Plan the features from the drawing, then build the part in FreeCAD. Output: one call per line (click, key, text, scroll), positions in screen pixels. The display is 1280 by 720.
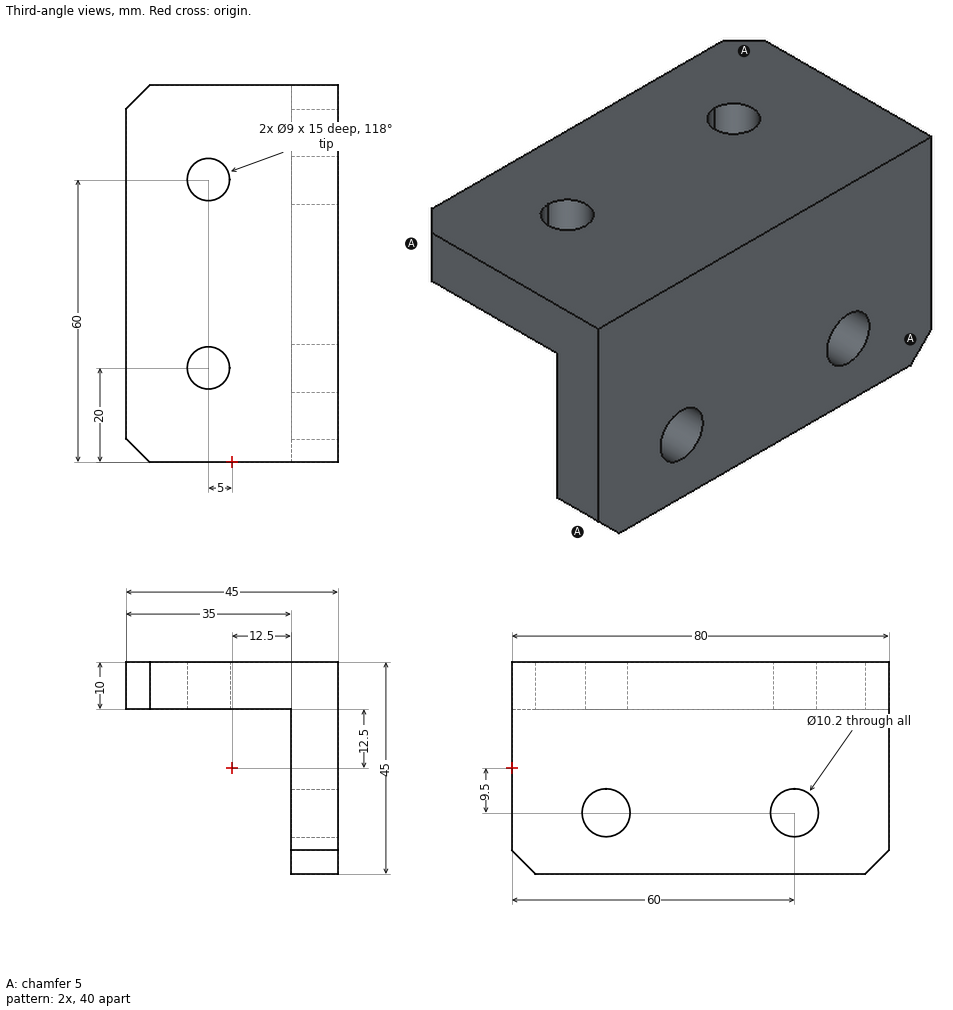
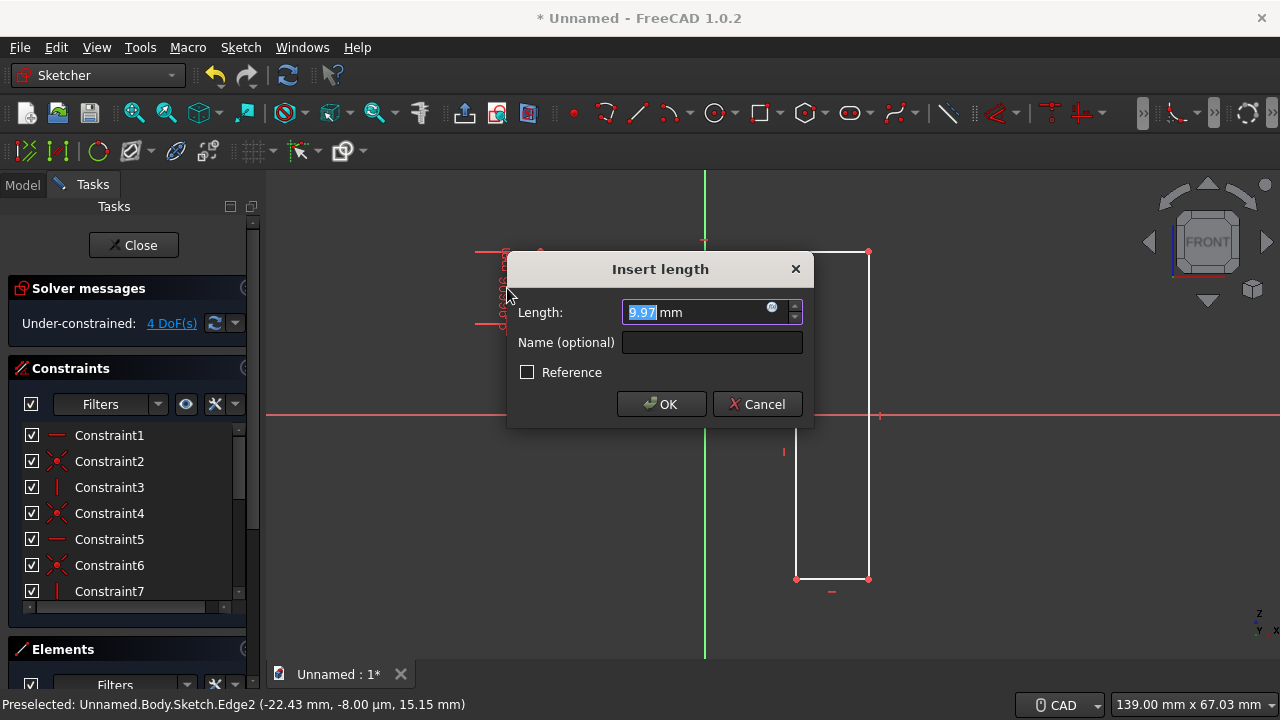
text(10)
key(Return)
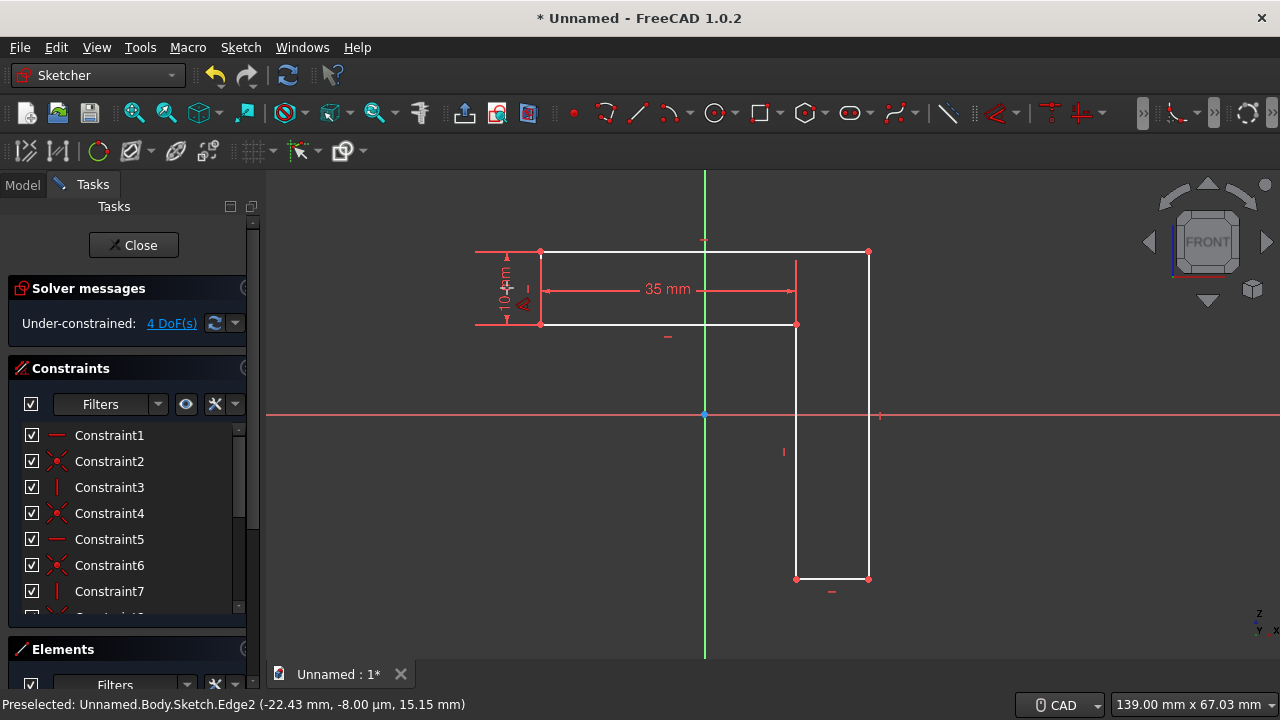
click(639, 252)
click(629, 218)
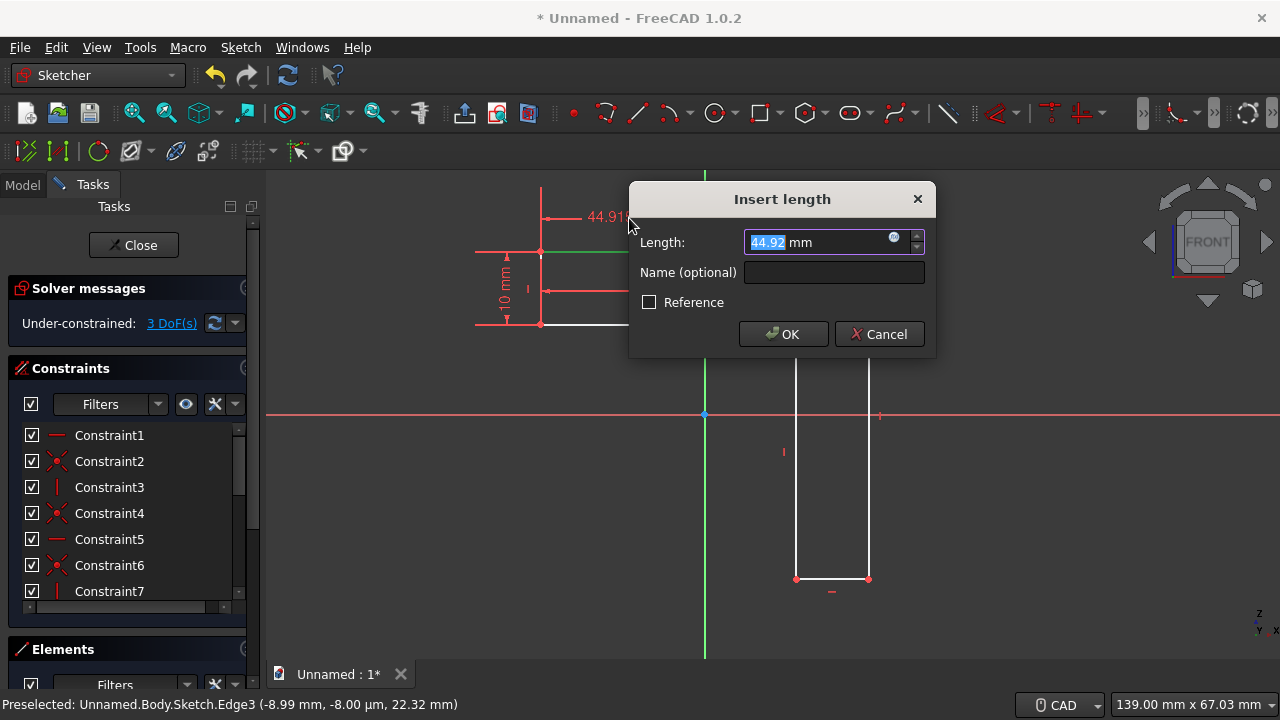
text(45)
key(Return)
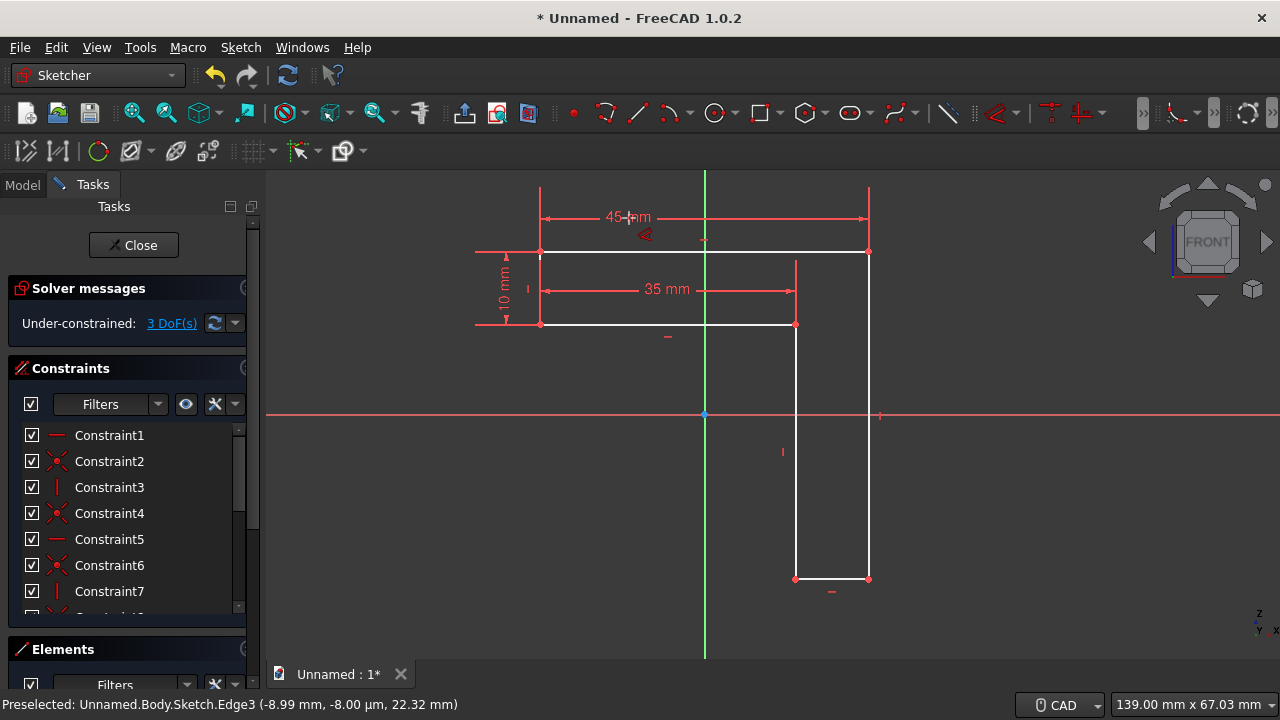
click(869, 350)
click(903, 340)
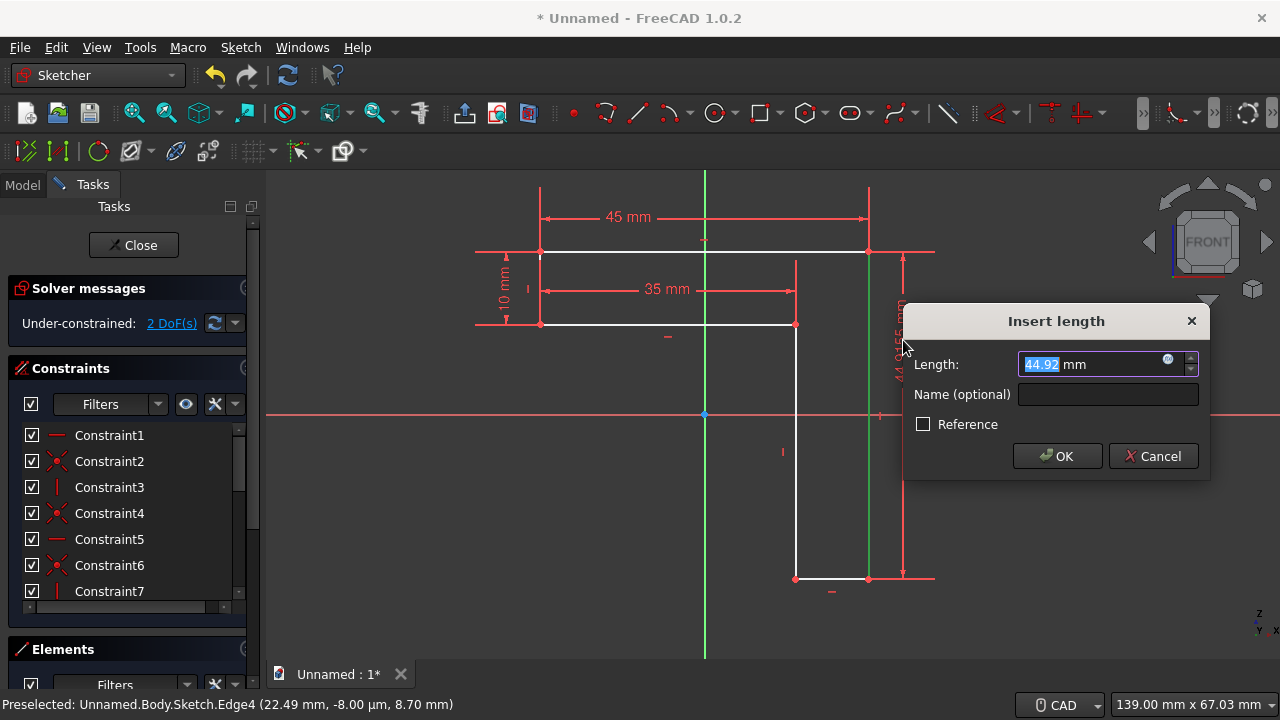
text(45)
key(Return)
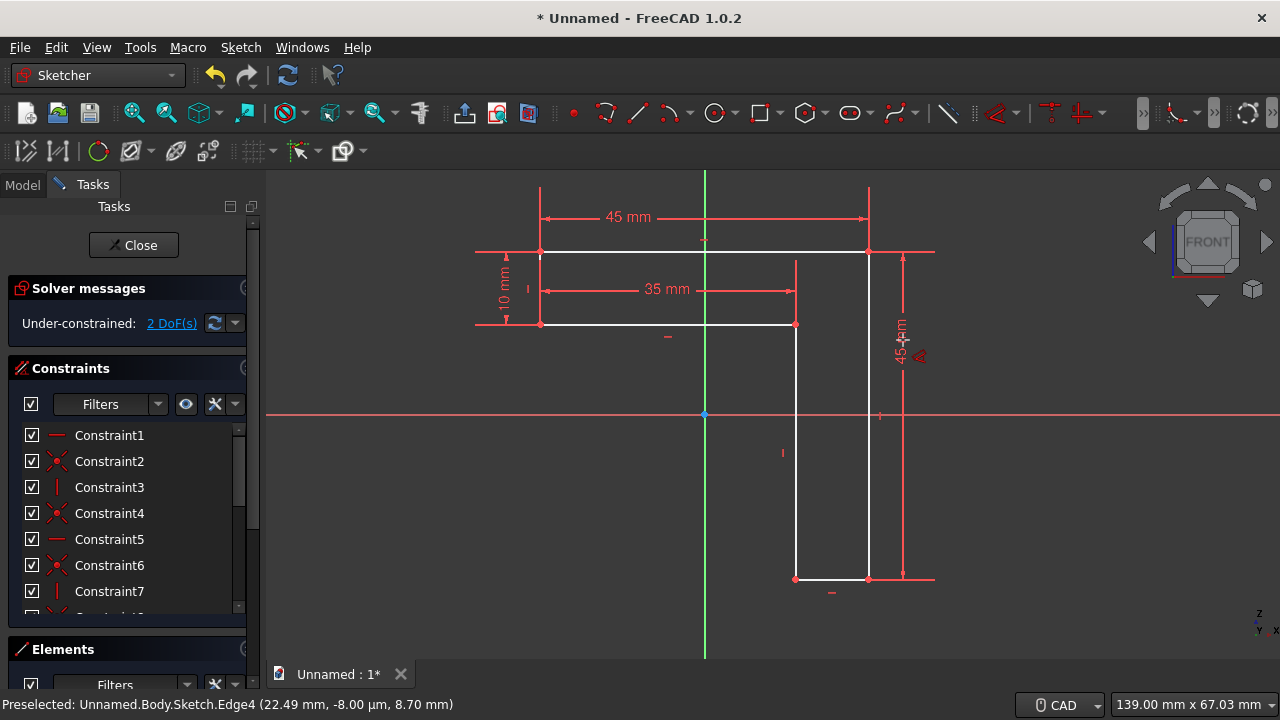
click(796, 325)
click(750, 291)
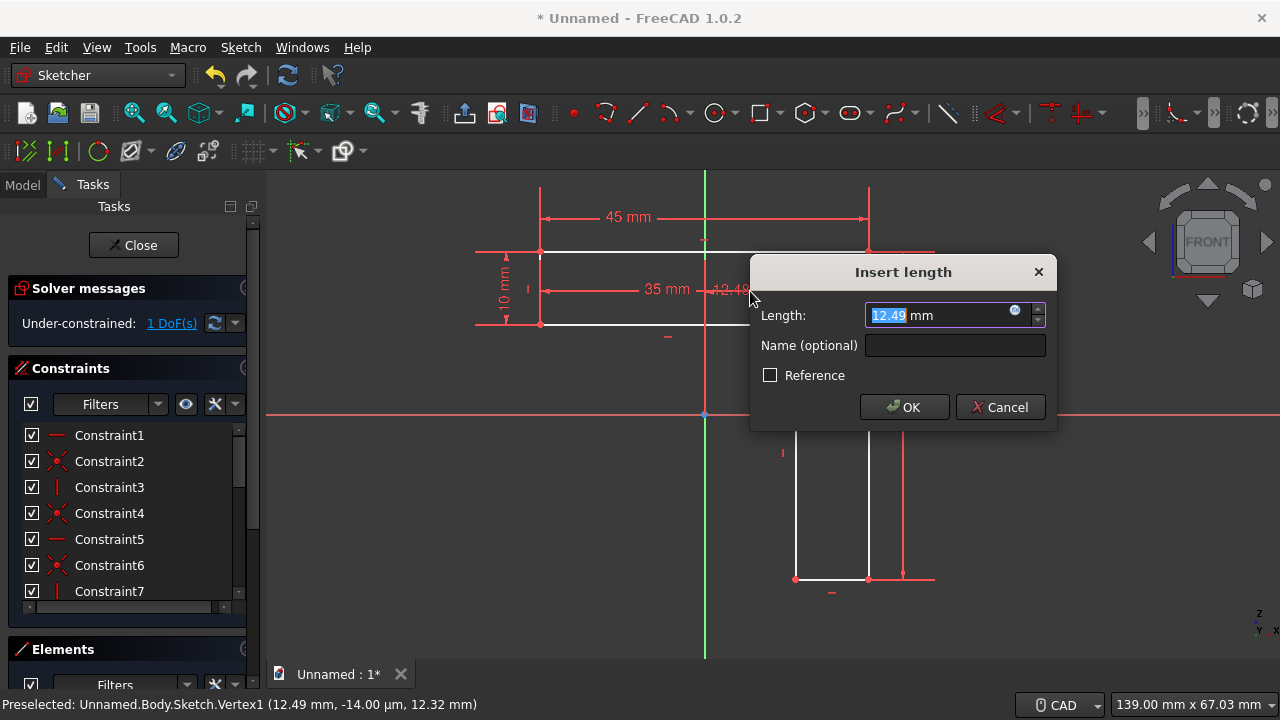
text(12.5)
key(Return)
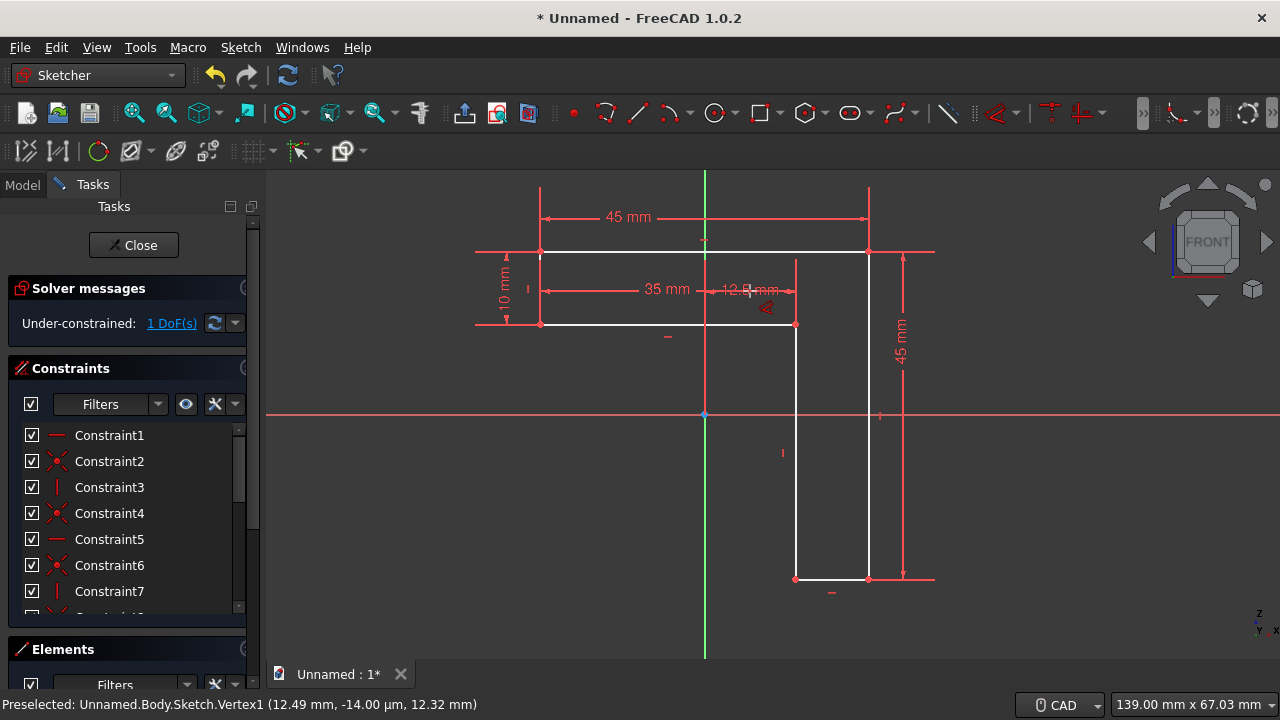
click(796, 325)
click(830, 370)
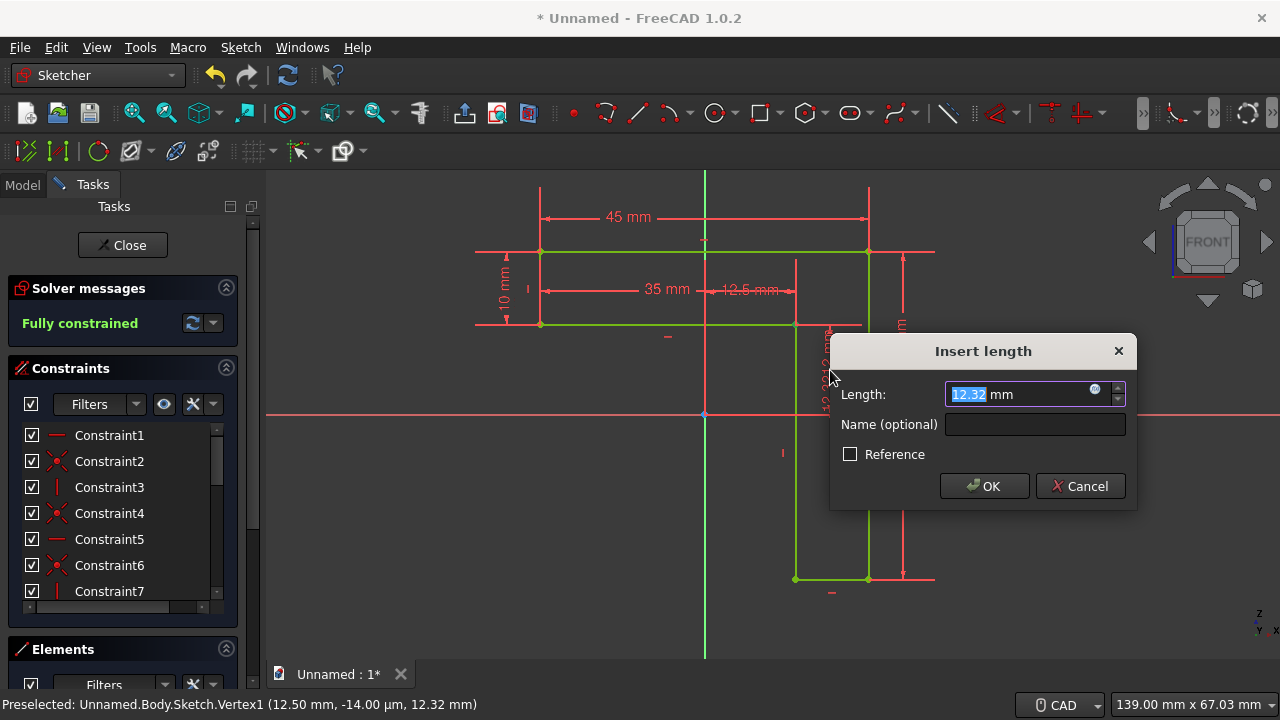
text(12.5)
key(Return)
key(Escape)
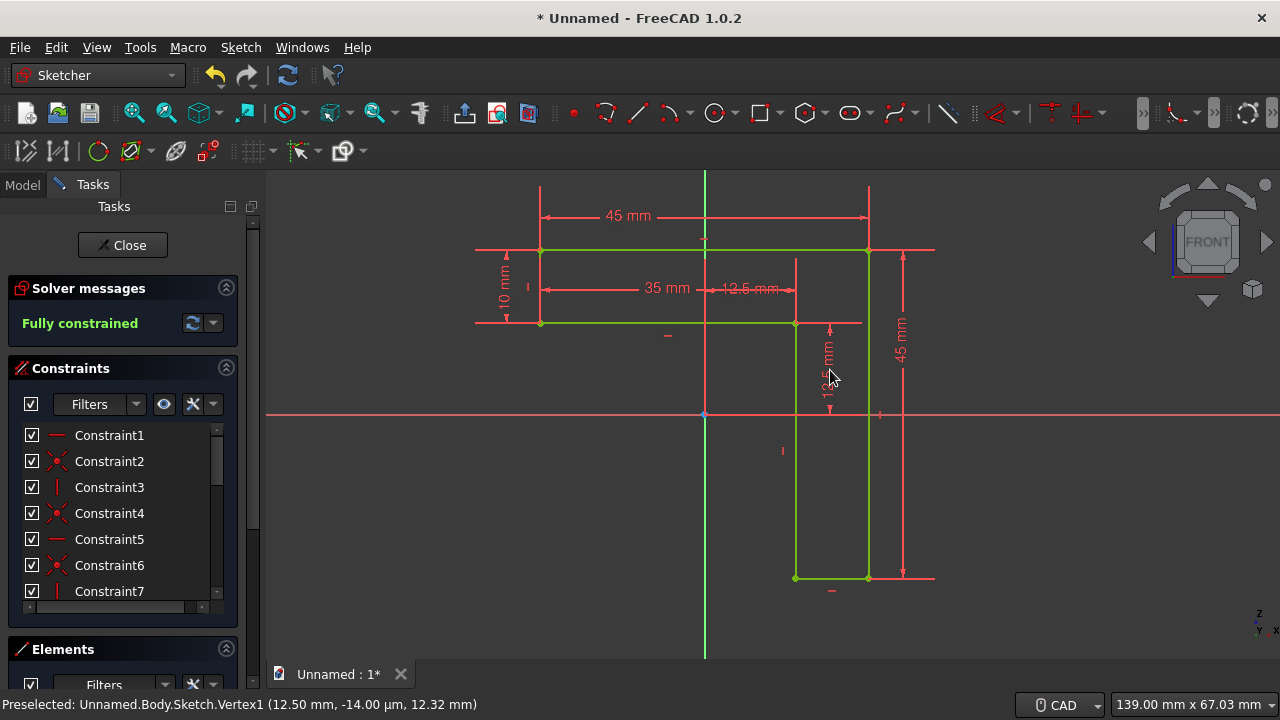
click(123, 245)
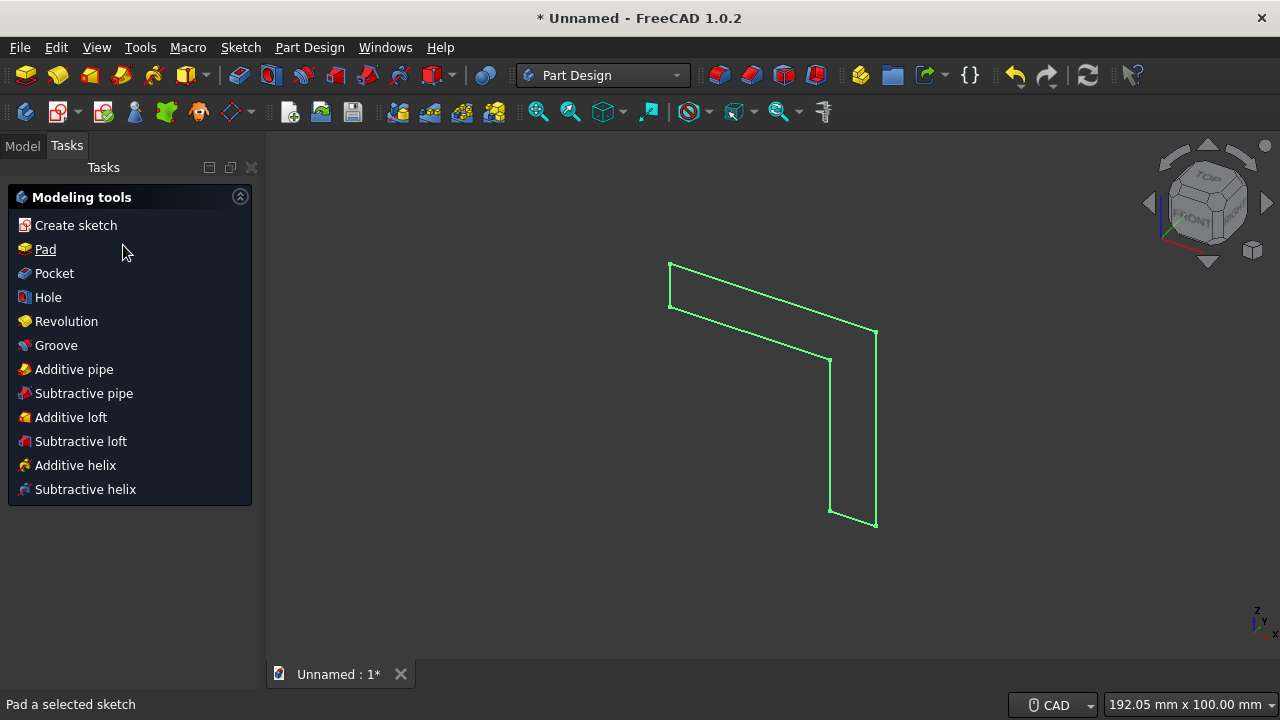
click(26, 76)